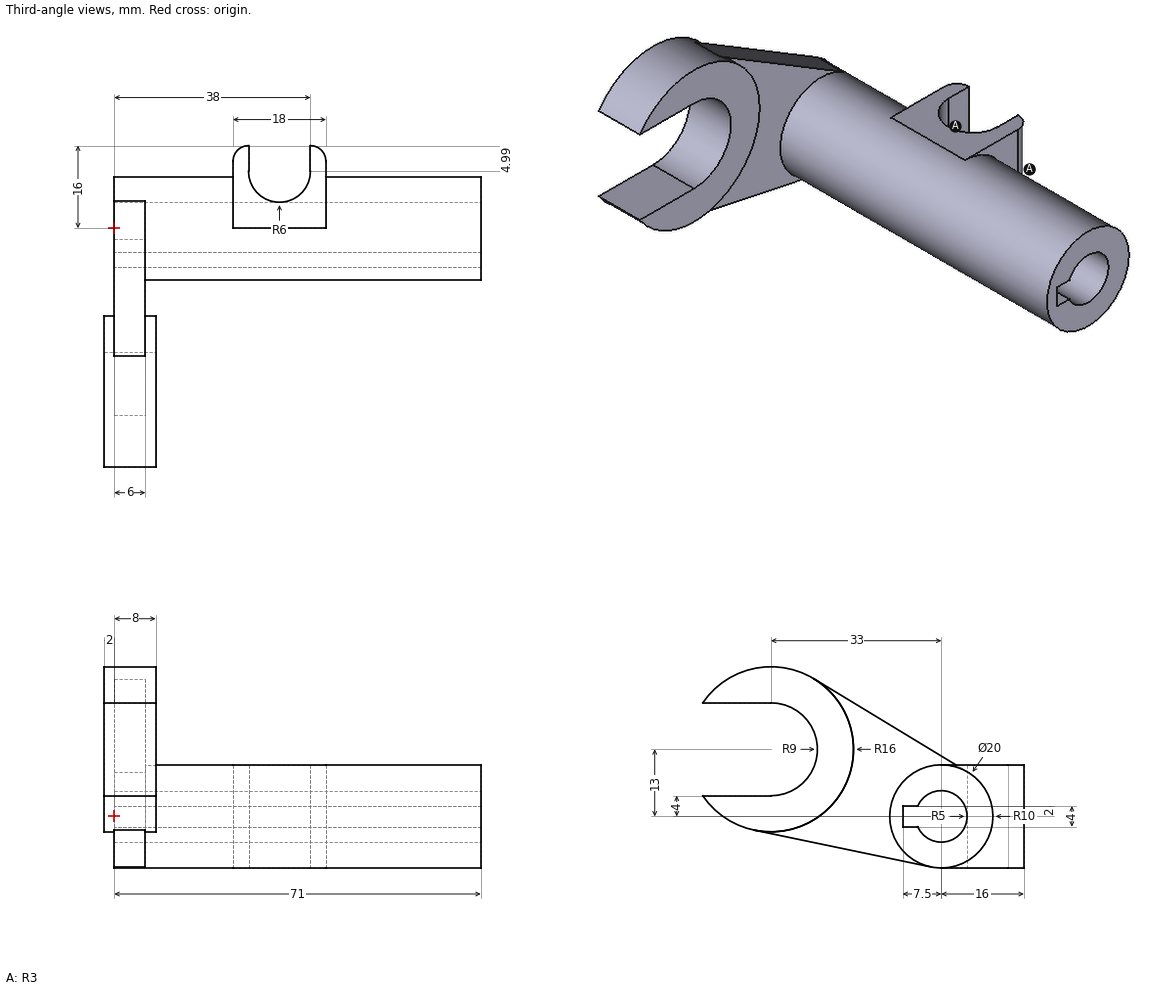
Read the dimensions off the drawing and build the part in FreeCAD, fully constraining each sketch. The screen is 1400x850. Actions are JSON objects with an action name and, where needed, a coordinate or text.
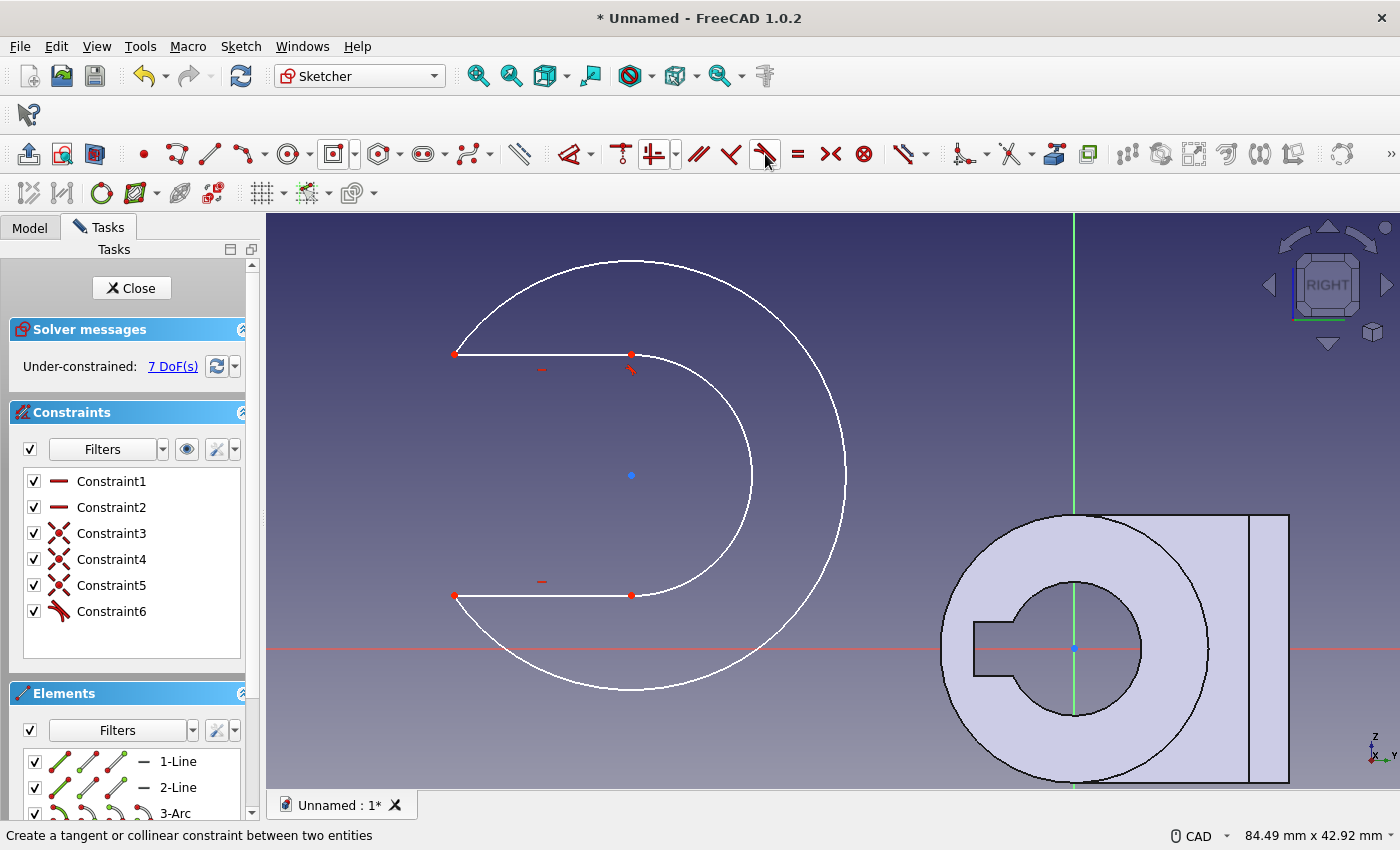
{"action": "left_click", "coordinate": [507, 596]}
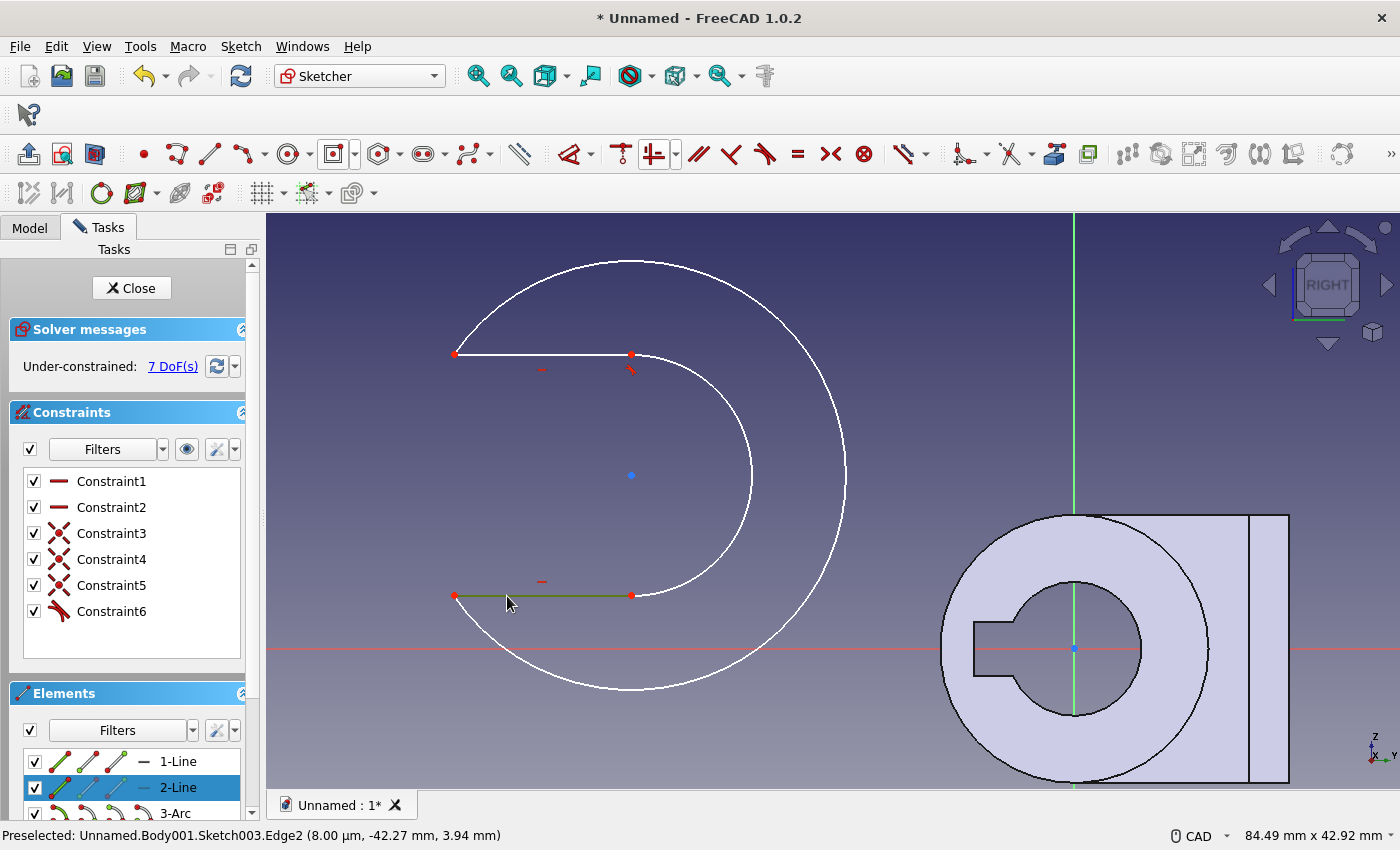
{"action": "left_click", "coordinate": [729, 547]}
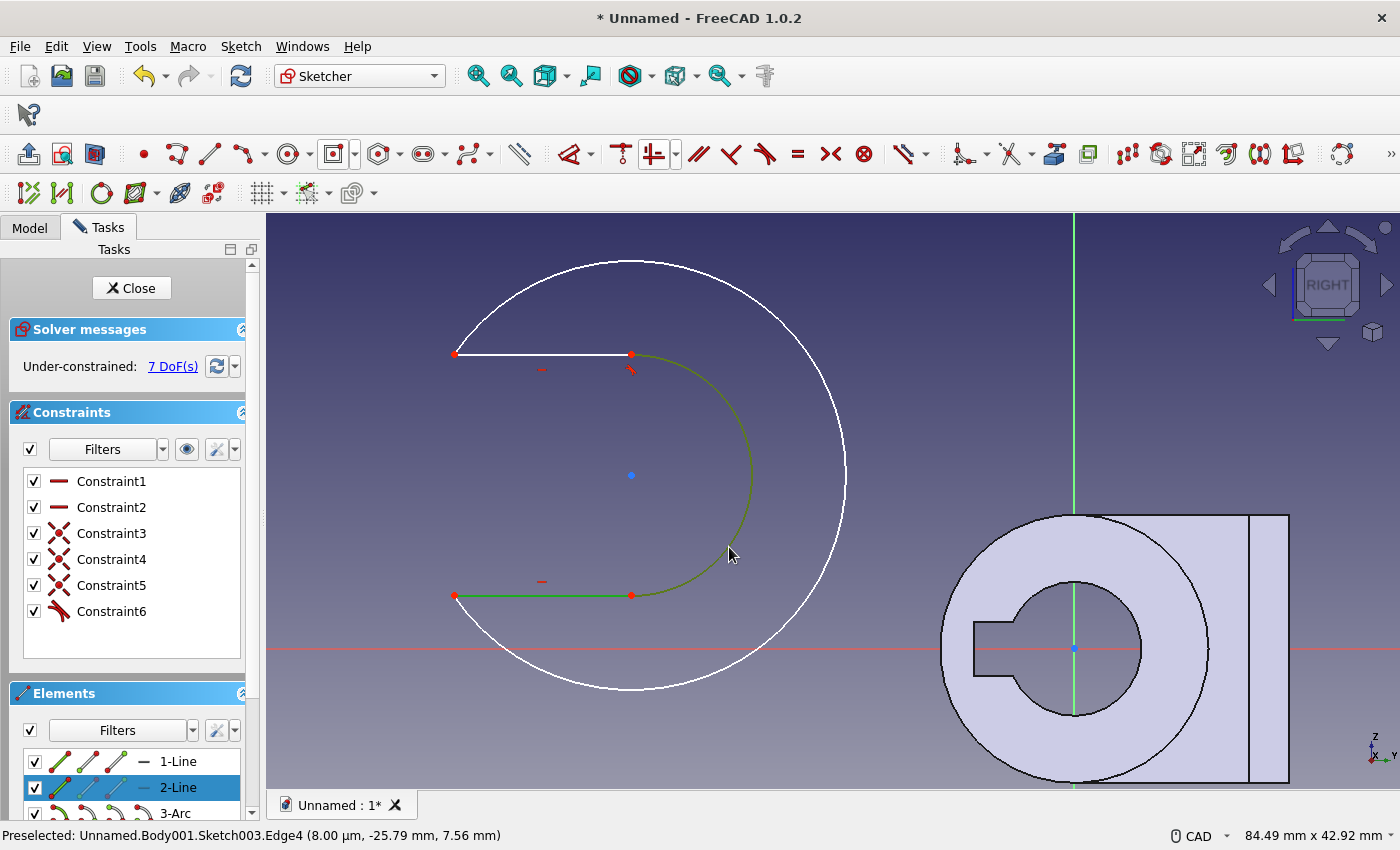
{"action": "key", "text": "t"}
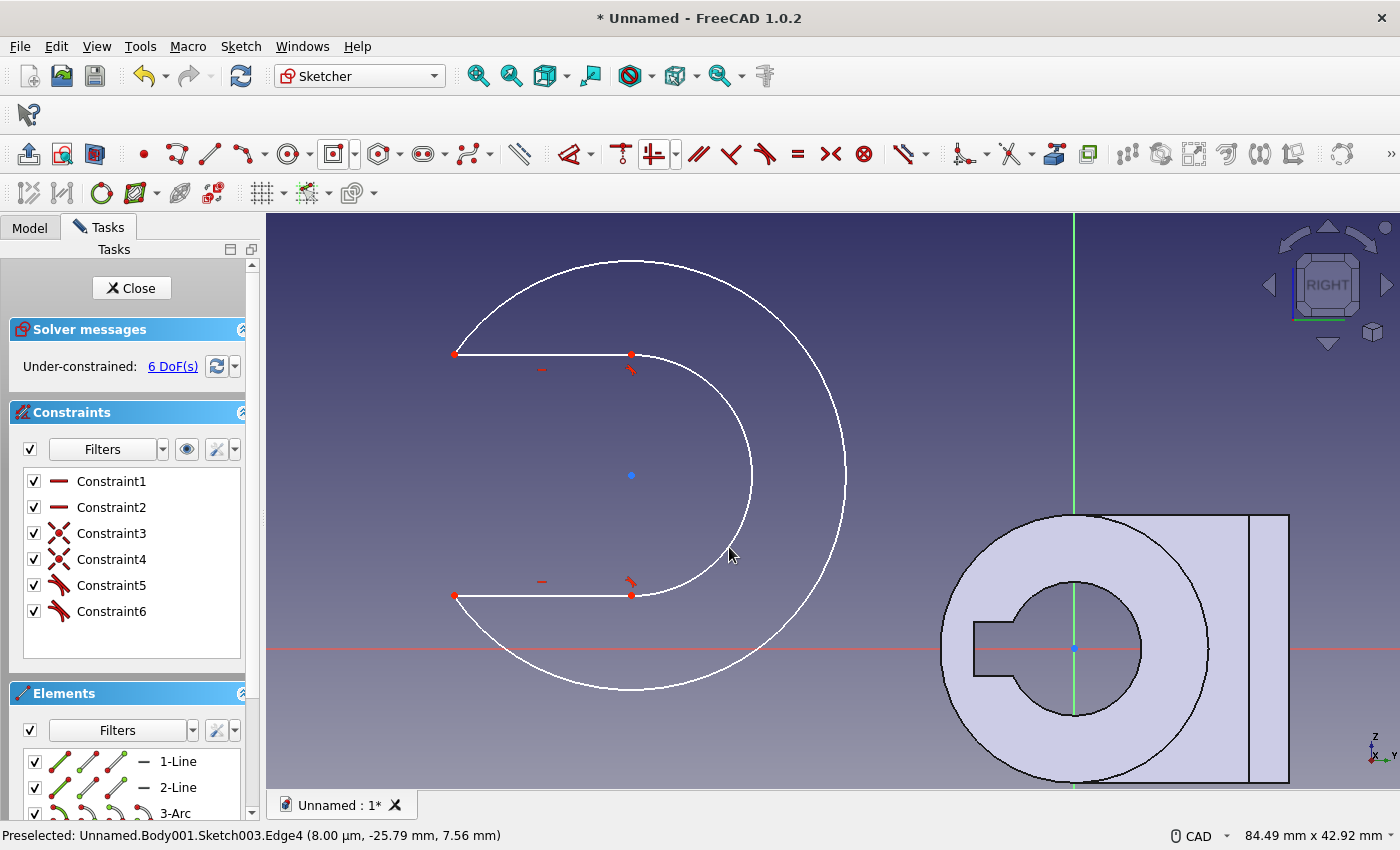
{"action": "scroll", "coordinate": [744, 658], "scroll_direction": "up", "scroll_amount": 3}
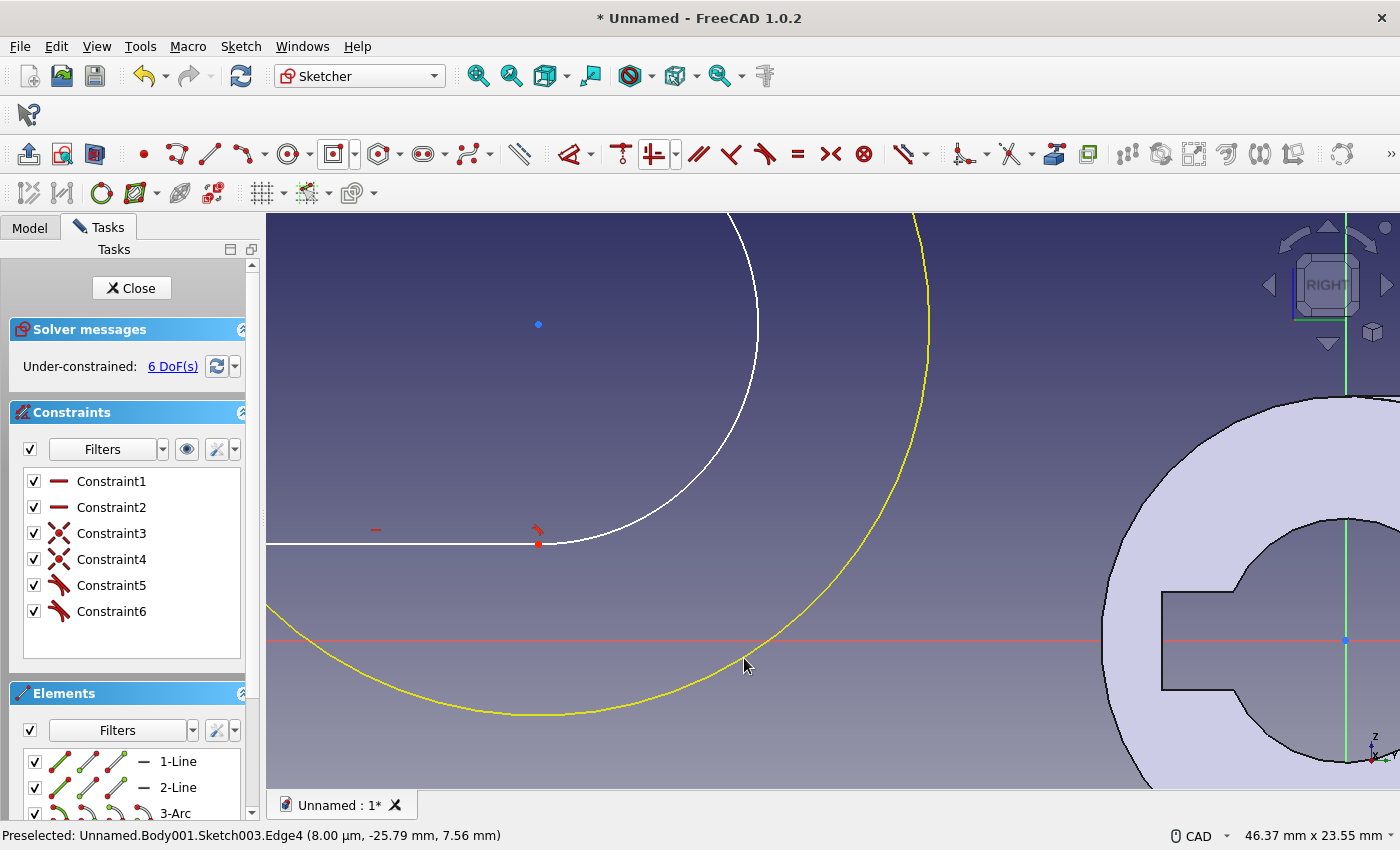
{"action": "left_click", "coordinate": [744, 658]}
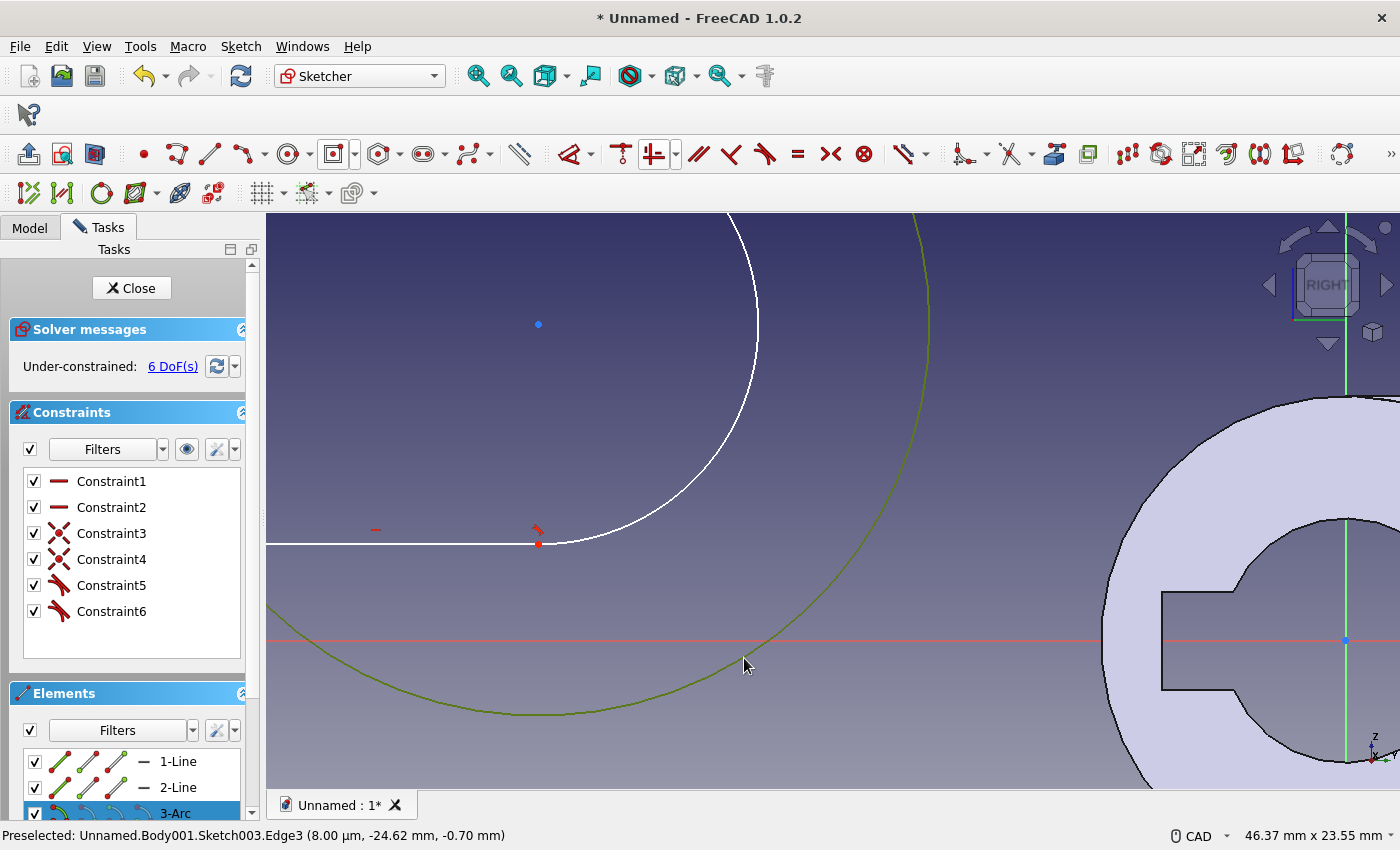
{"action": "left_click", "coordinate": [716, 454]}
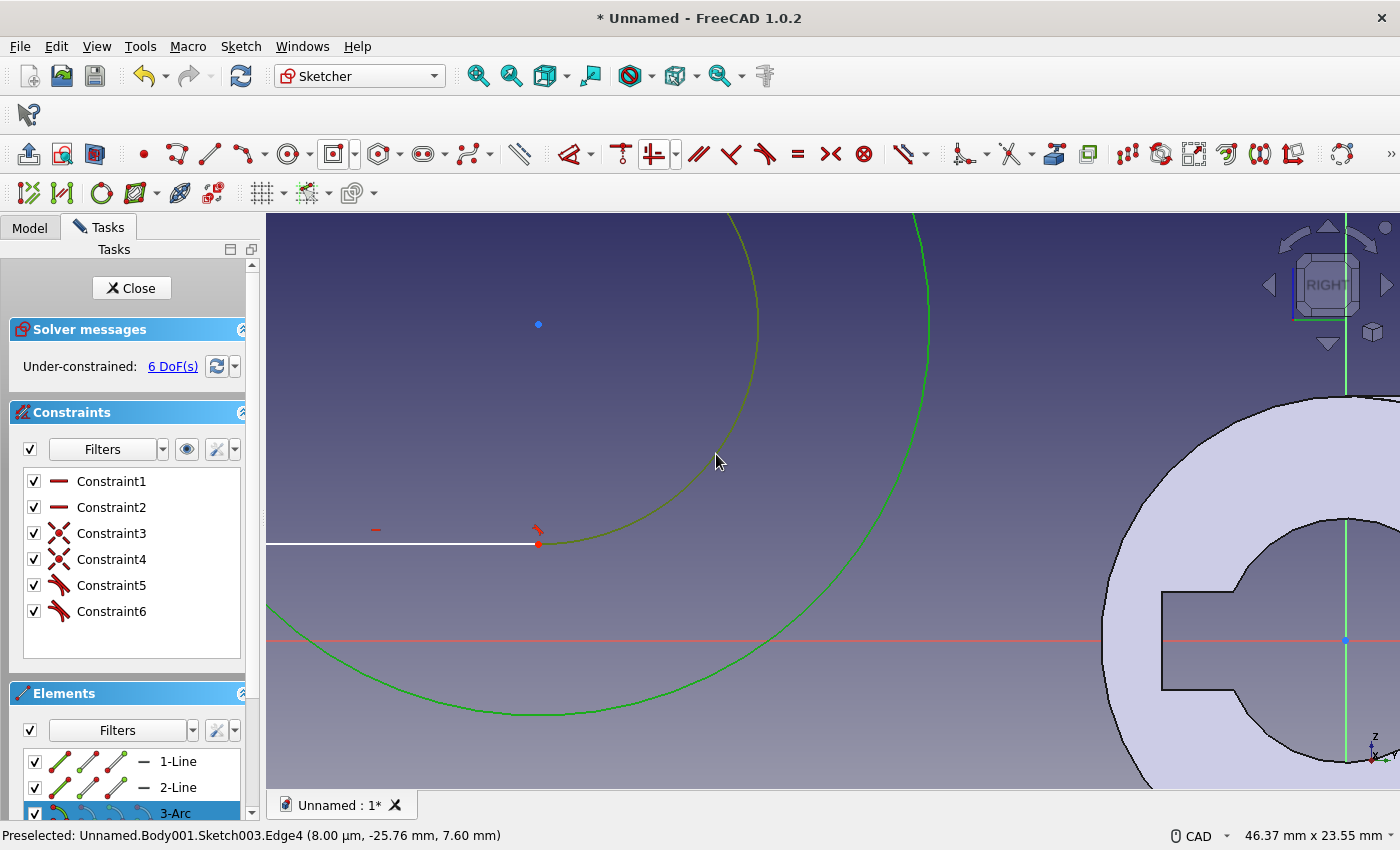
{"action": "key", "text": "c"}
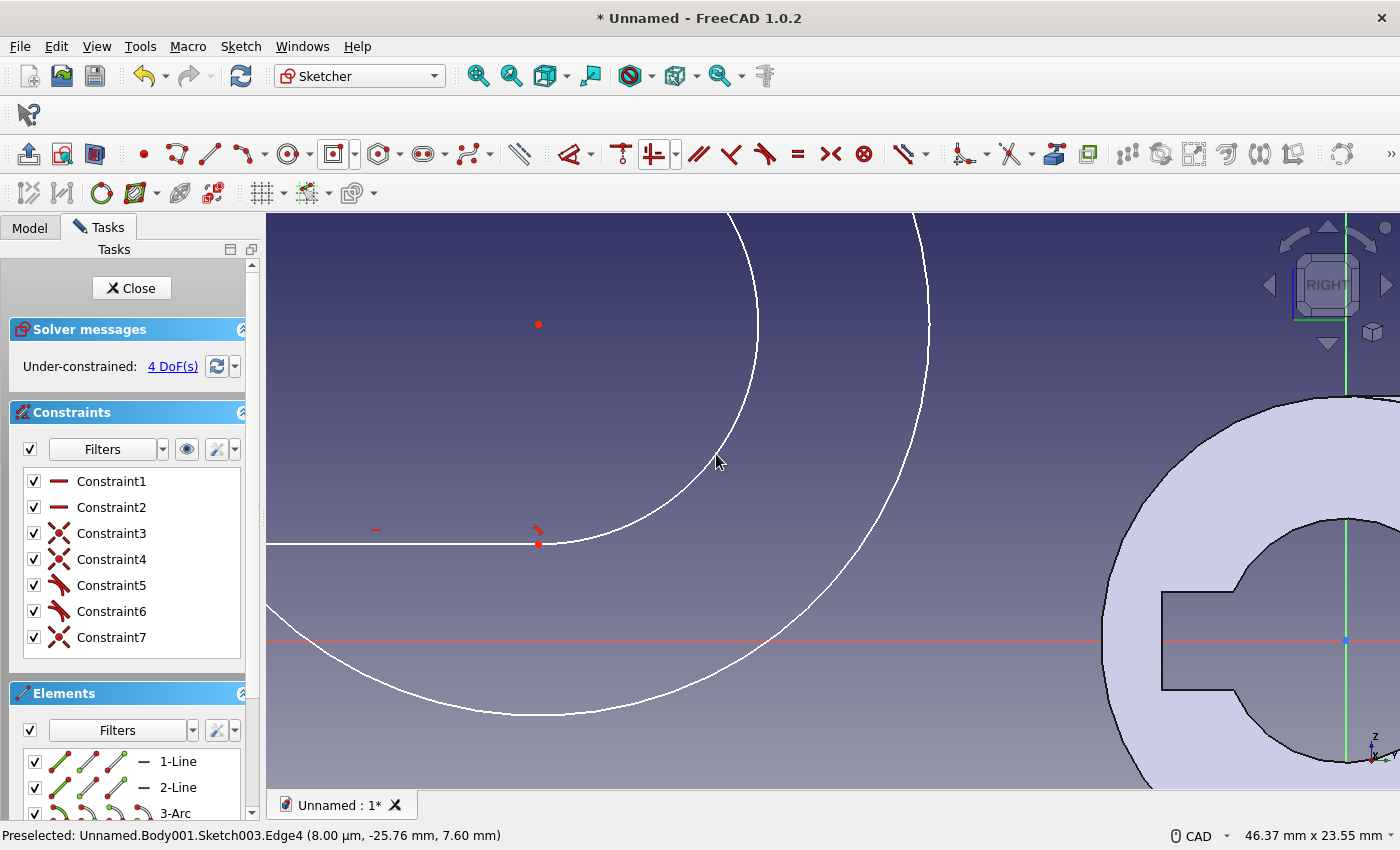
{"action": "left_click", "coordinate": [568, 154]}